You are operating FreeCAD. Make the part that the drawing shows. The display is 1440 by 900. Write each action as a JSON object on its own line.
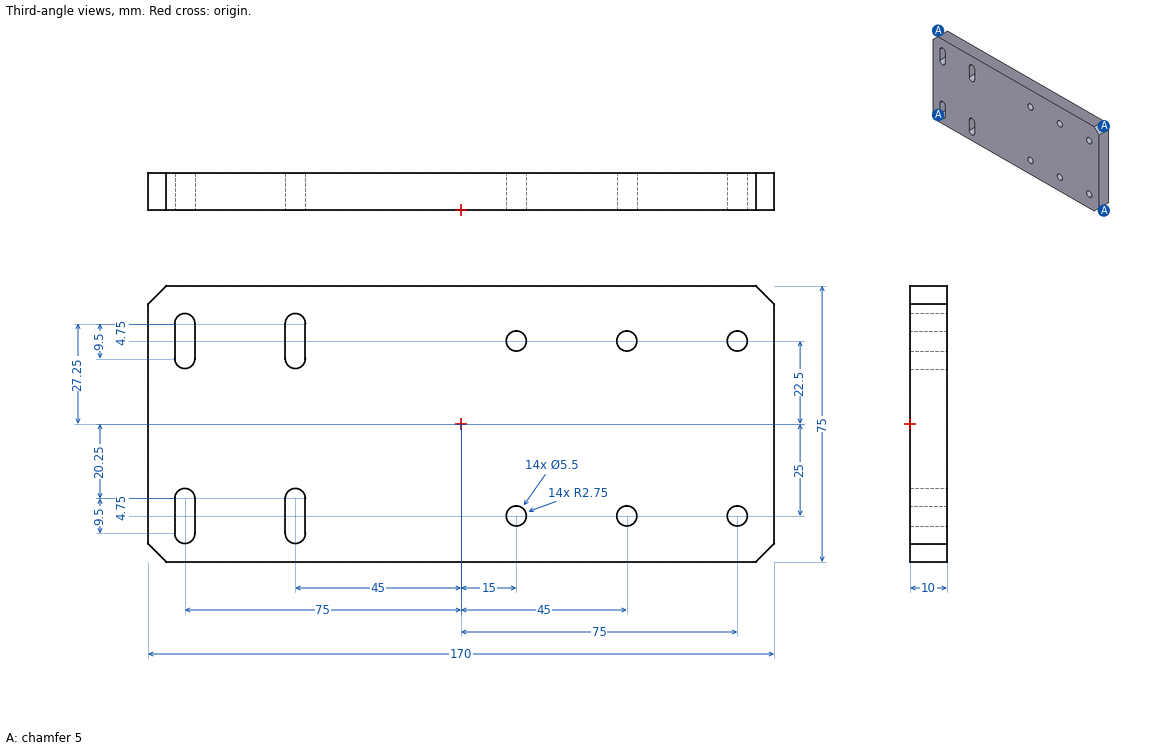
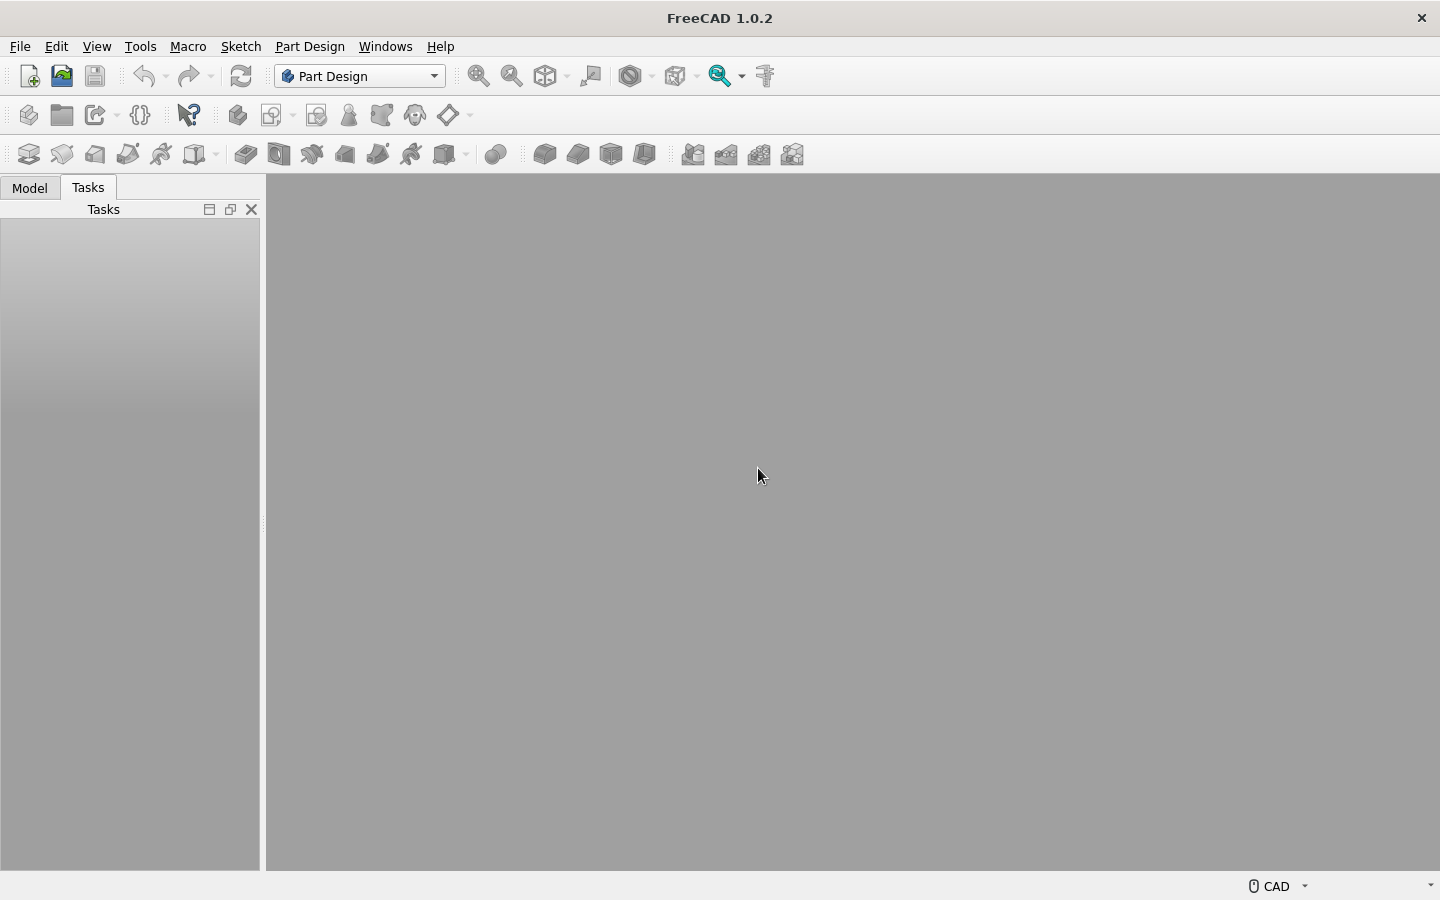
{"action": "key", "text": "ctrl+n"}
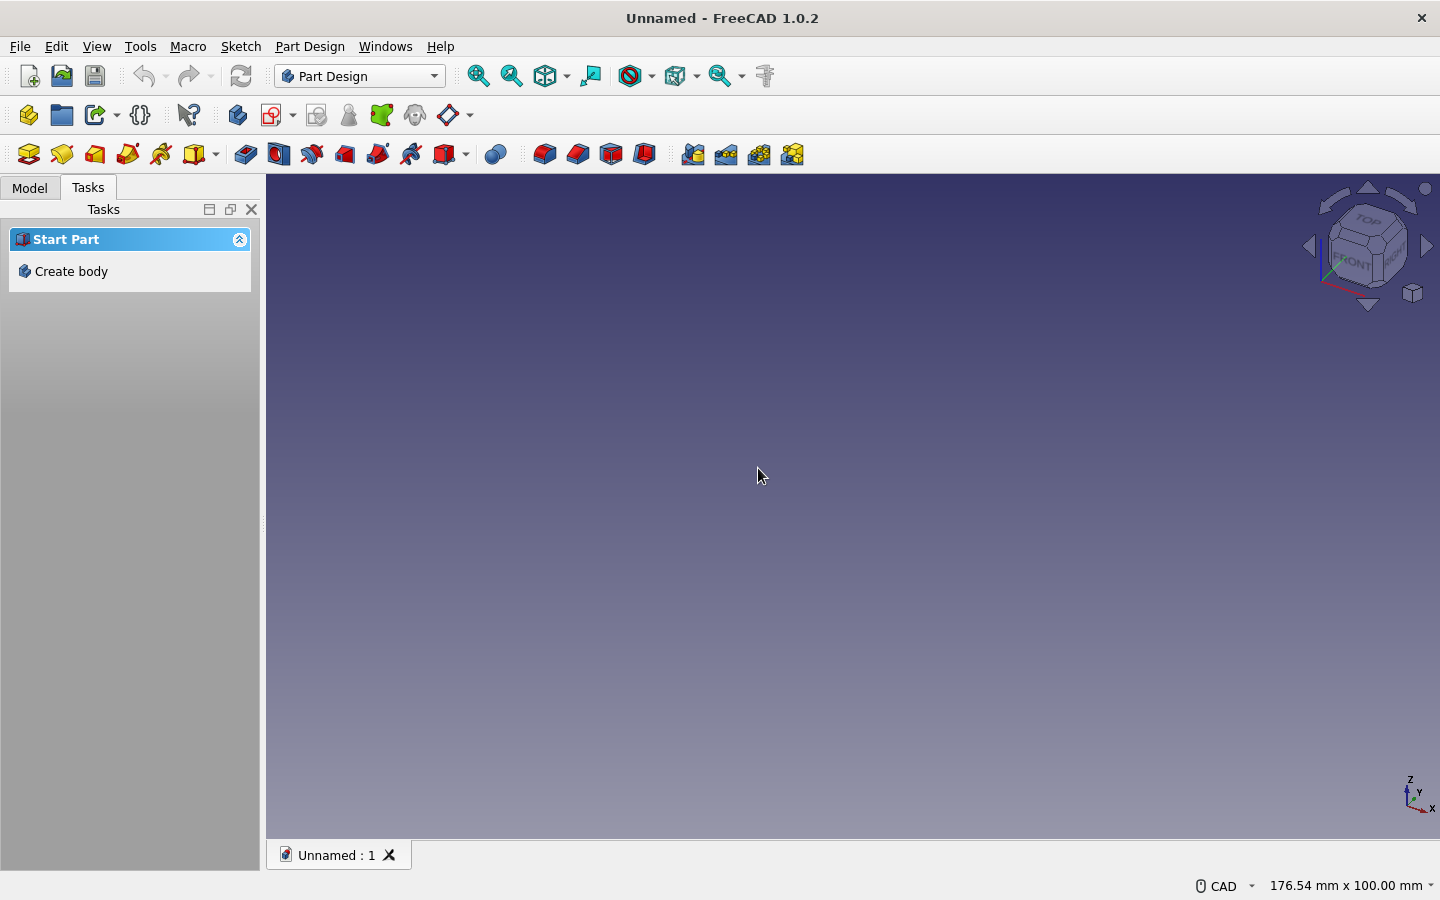
{"action": "left_click", "coordinate": [270, 116]}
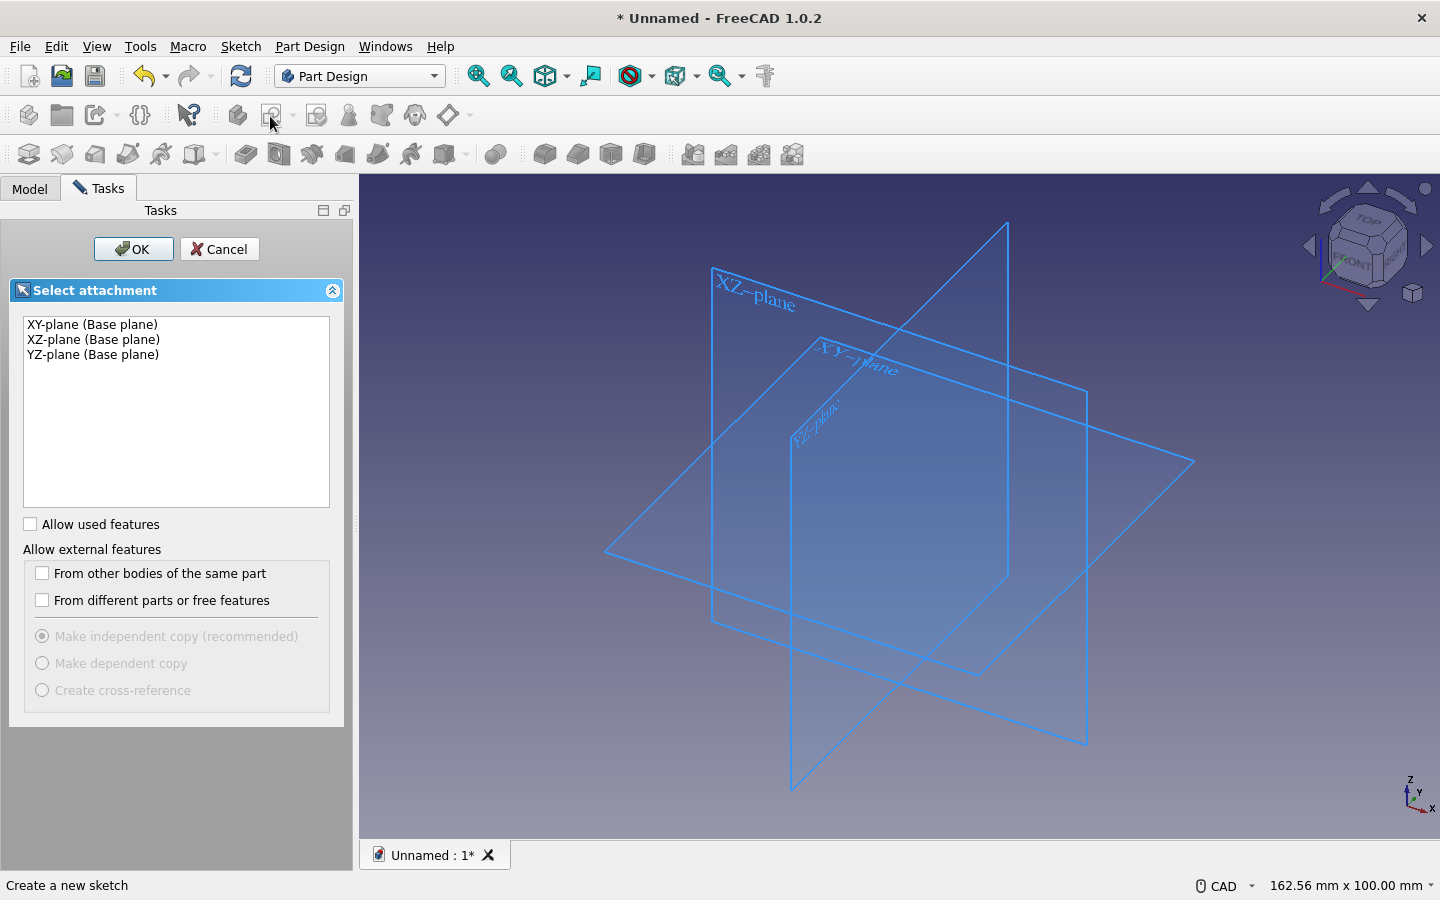
{"action": "left_click", "coordinate": [84, 340]}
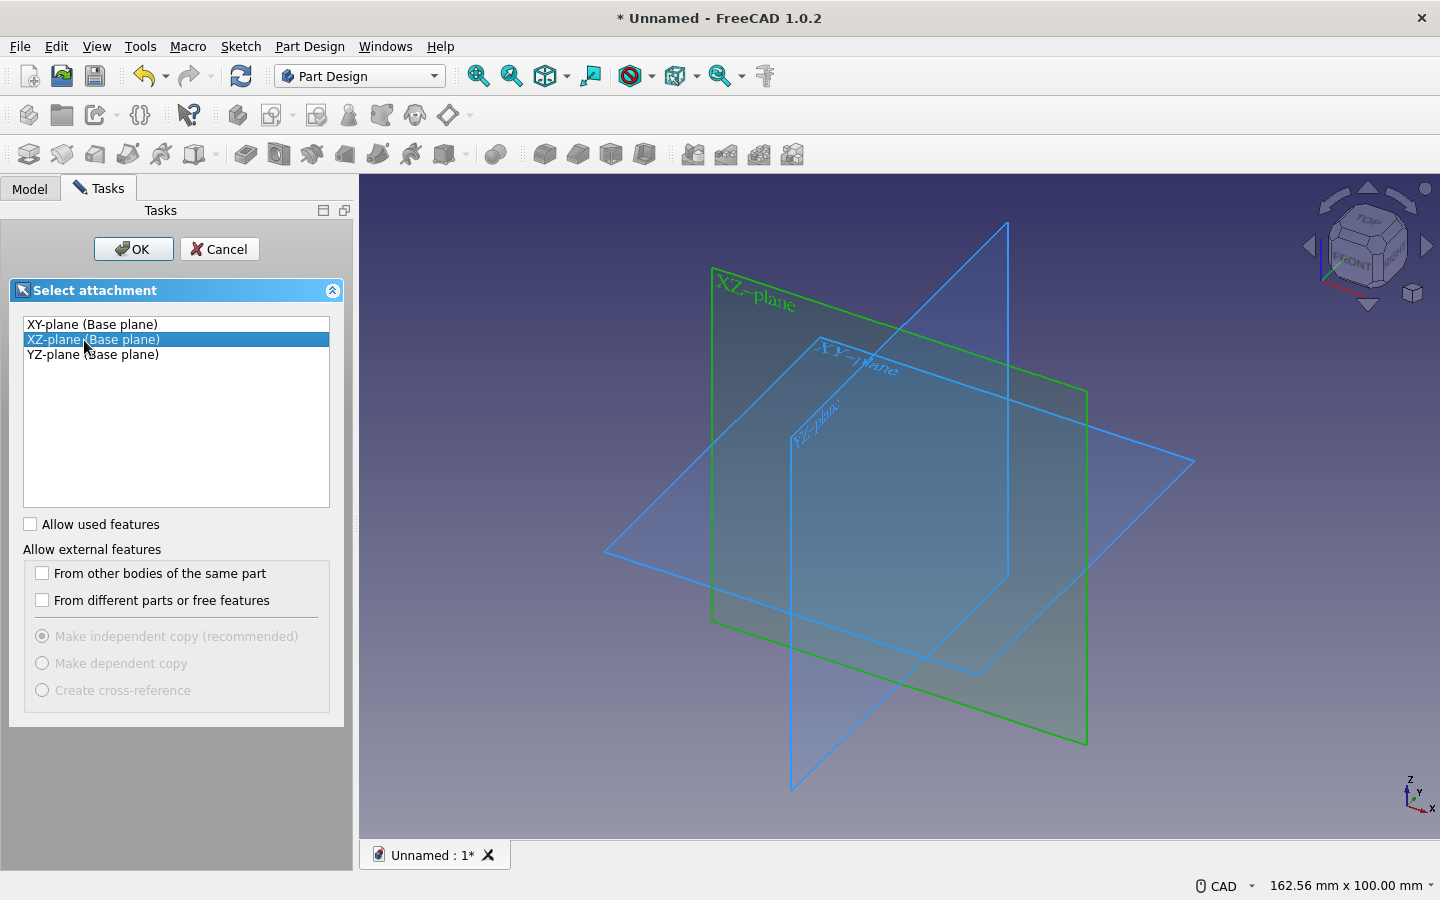
{"action": "left_click", "coordinate": [134, 249]}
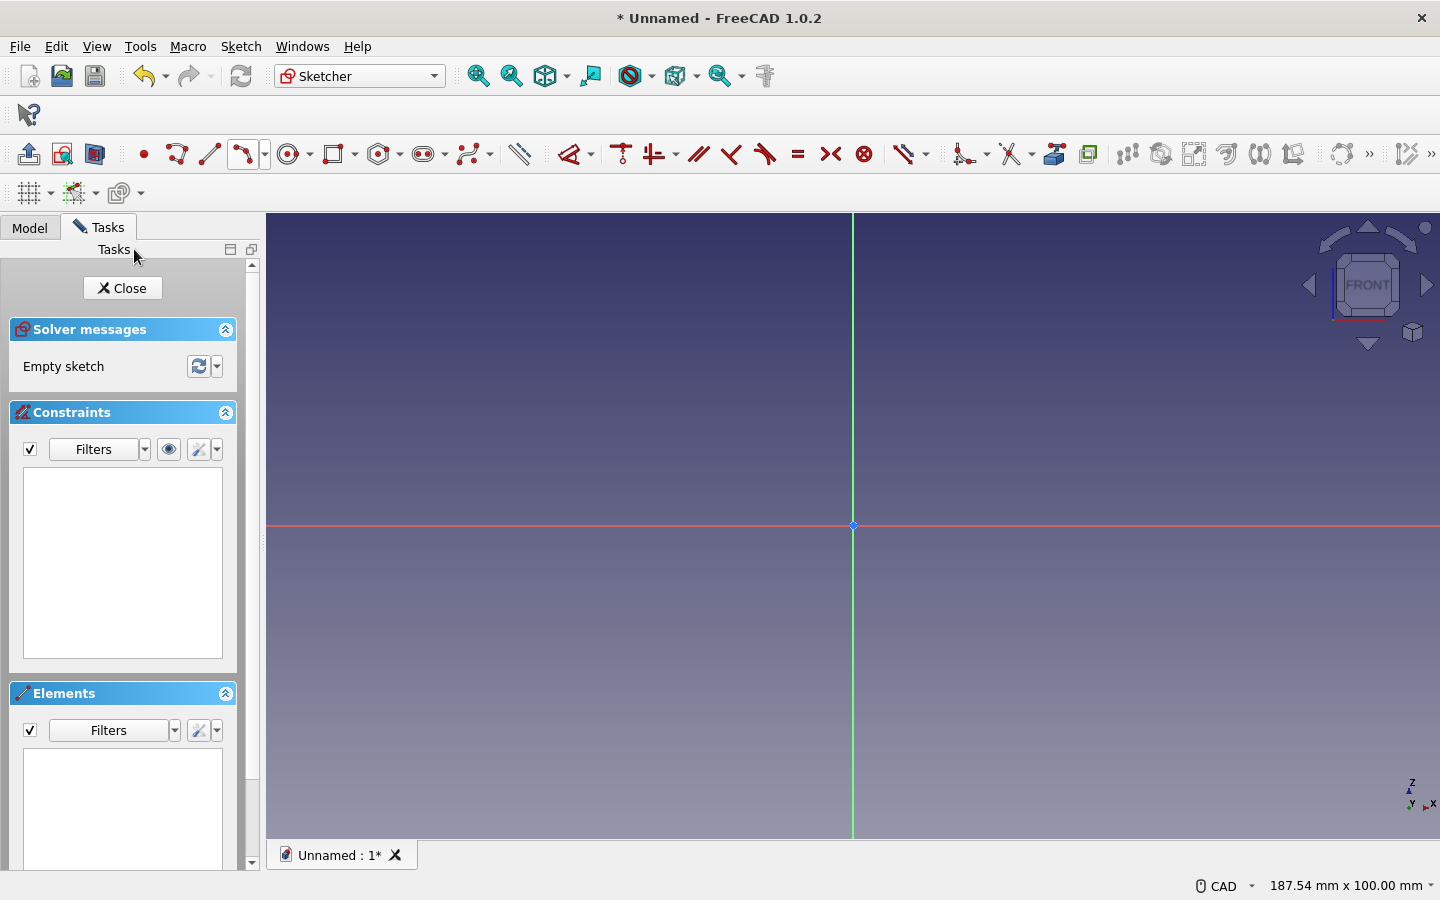
{"action": "scroll", "coordinate": [645, 526], "scroll_direction": "down", "scroll_amount": 2}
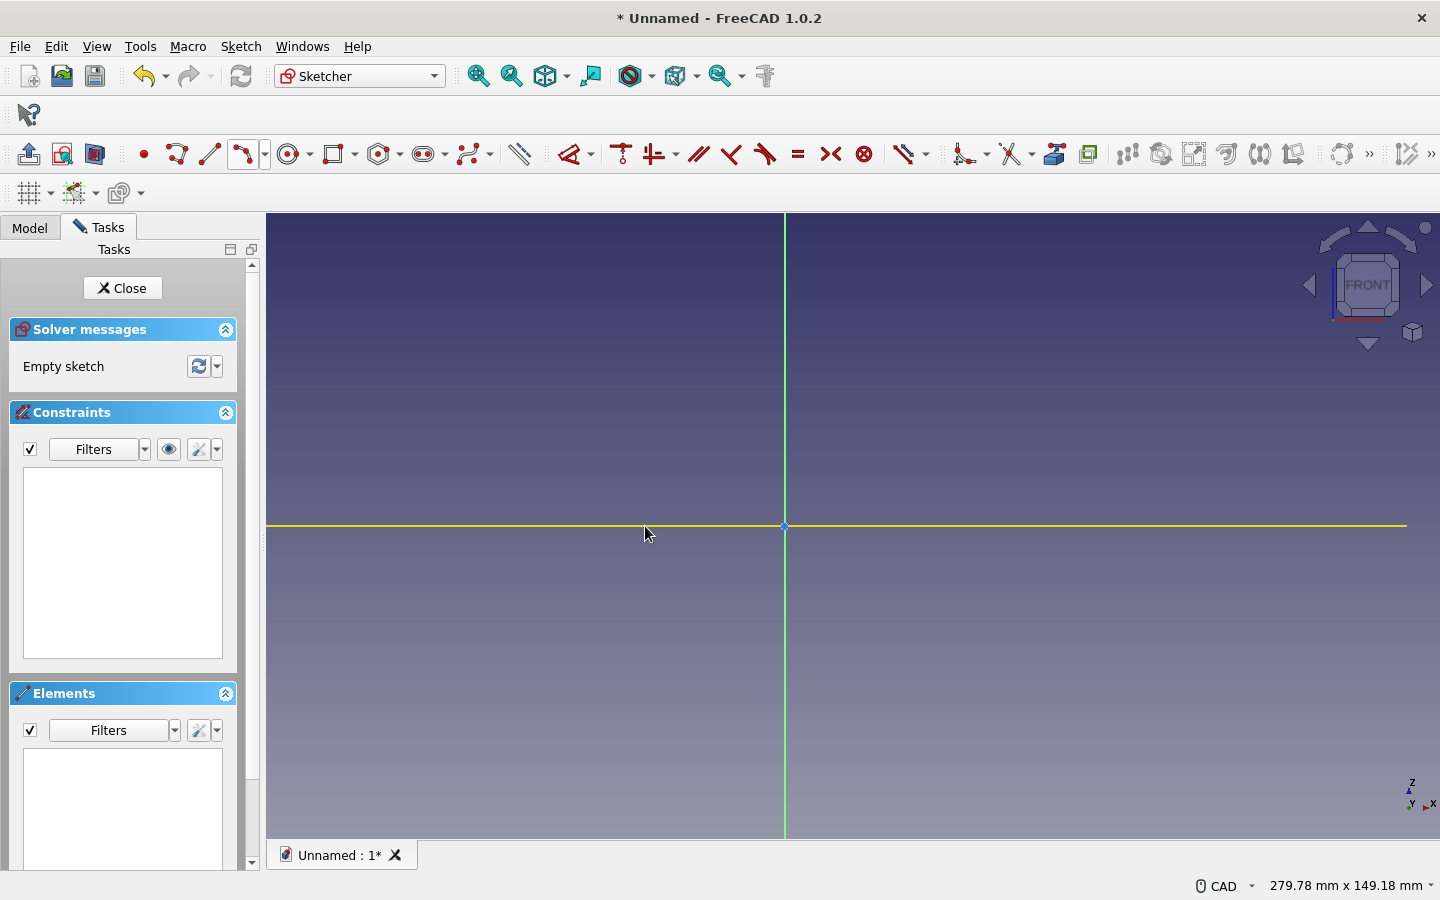
{"action": "key", "text": "g v"}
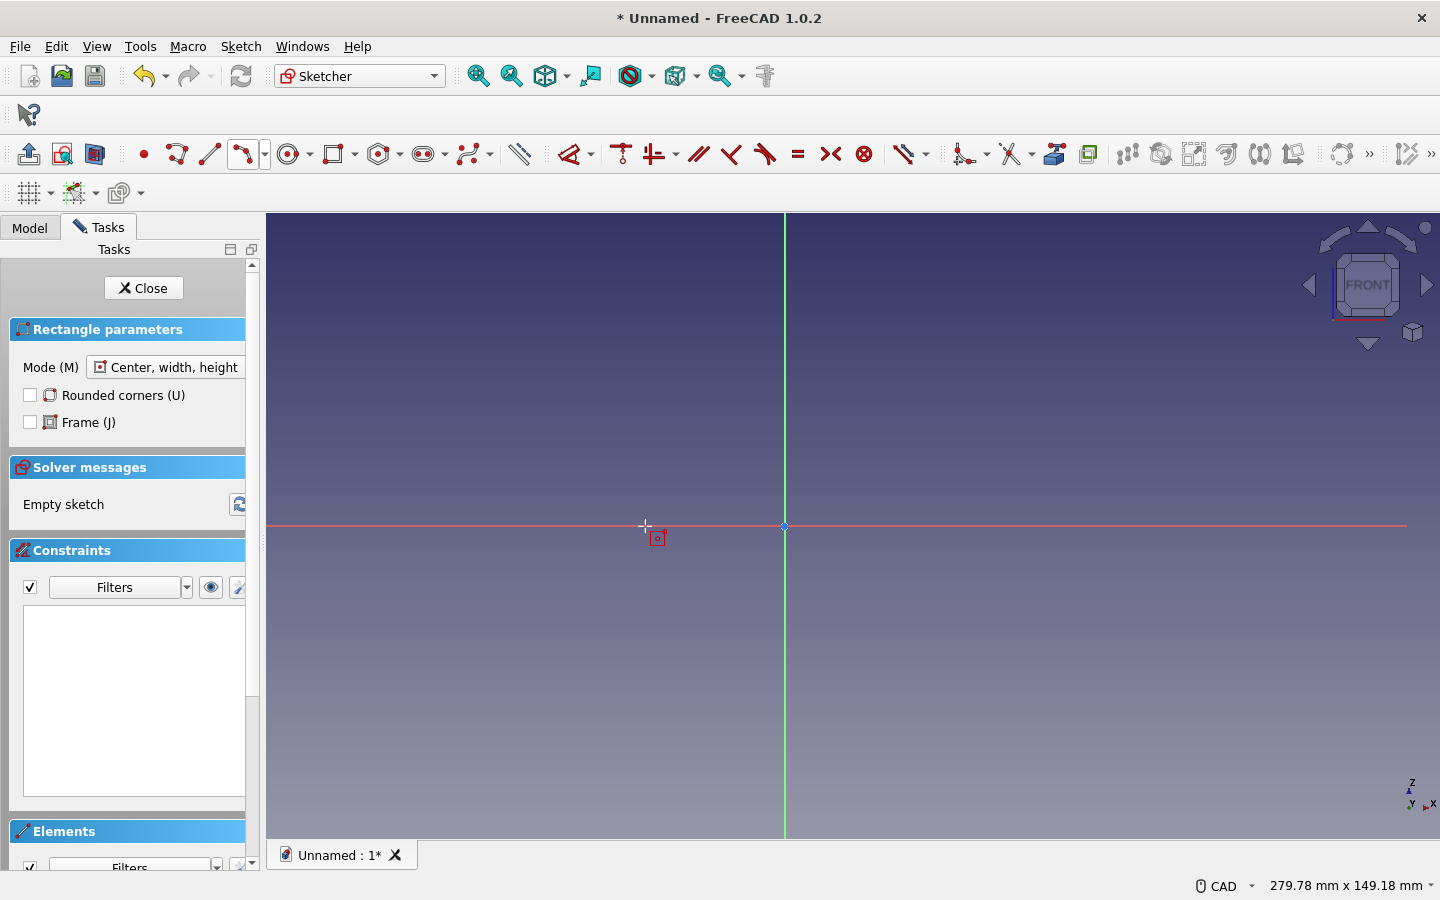
{"action": "left_click", "coordinate": [785, 526]}
{"action": "left_click", "coordinate": [1141, 369]}
{"action": "key", "text": "Escape"}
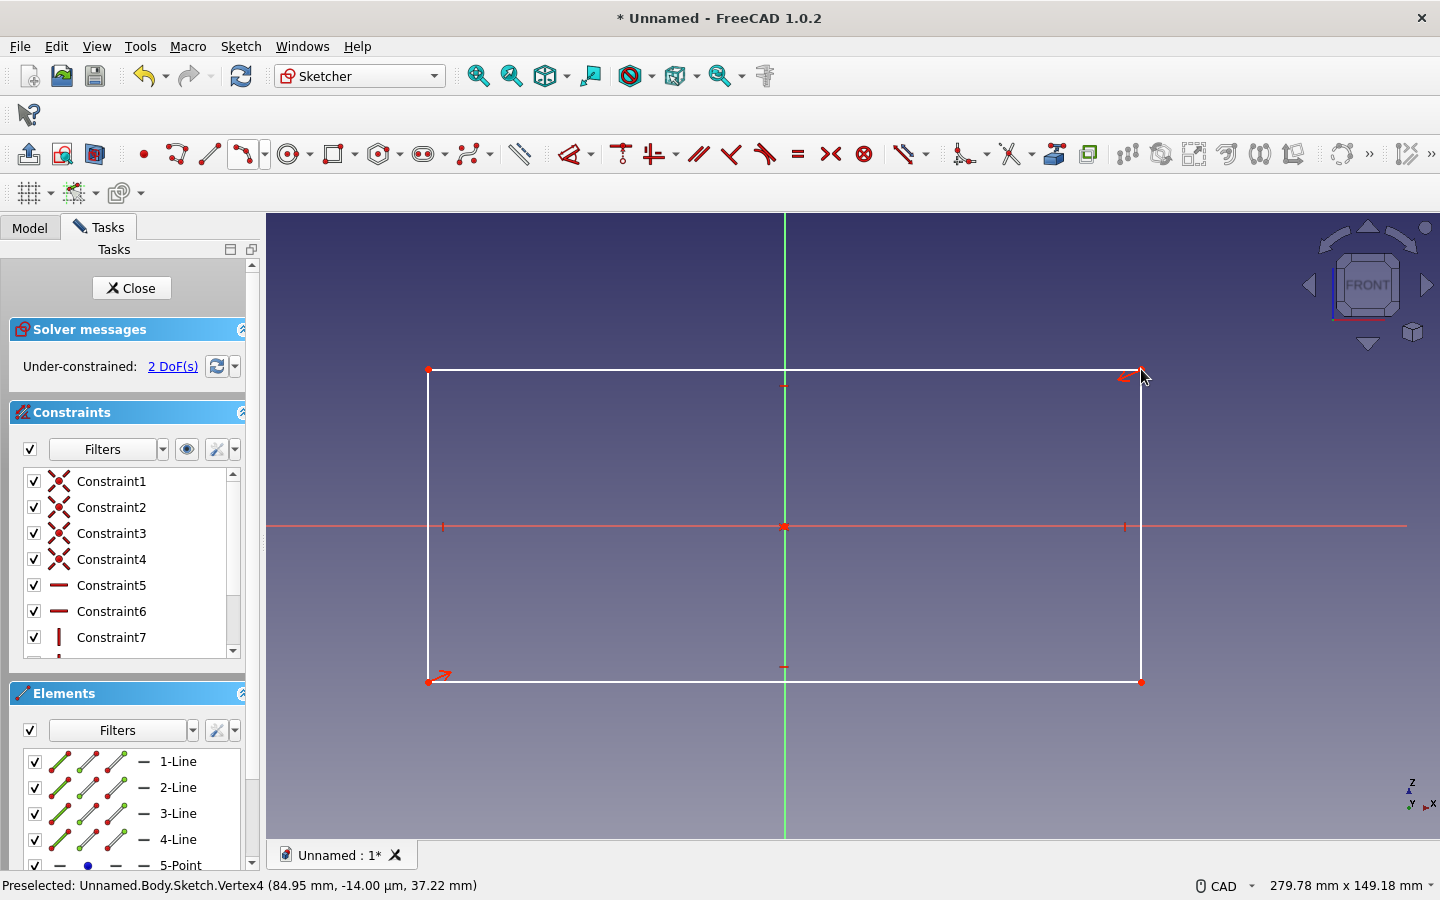
{"action": "left_click", "coordinate": [568, 154]}